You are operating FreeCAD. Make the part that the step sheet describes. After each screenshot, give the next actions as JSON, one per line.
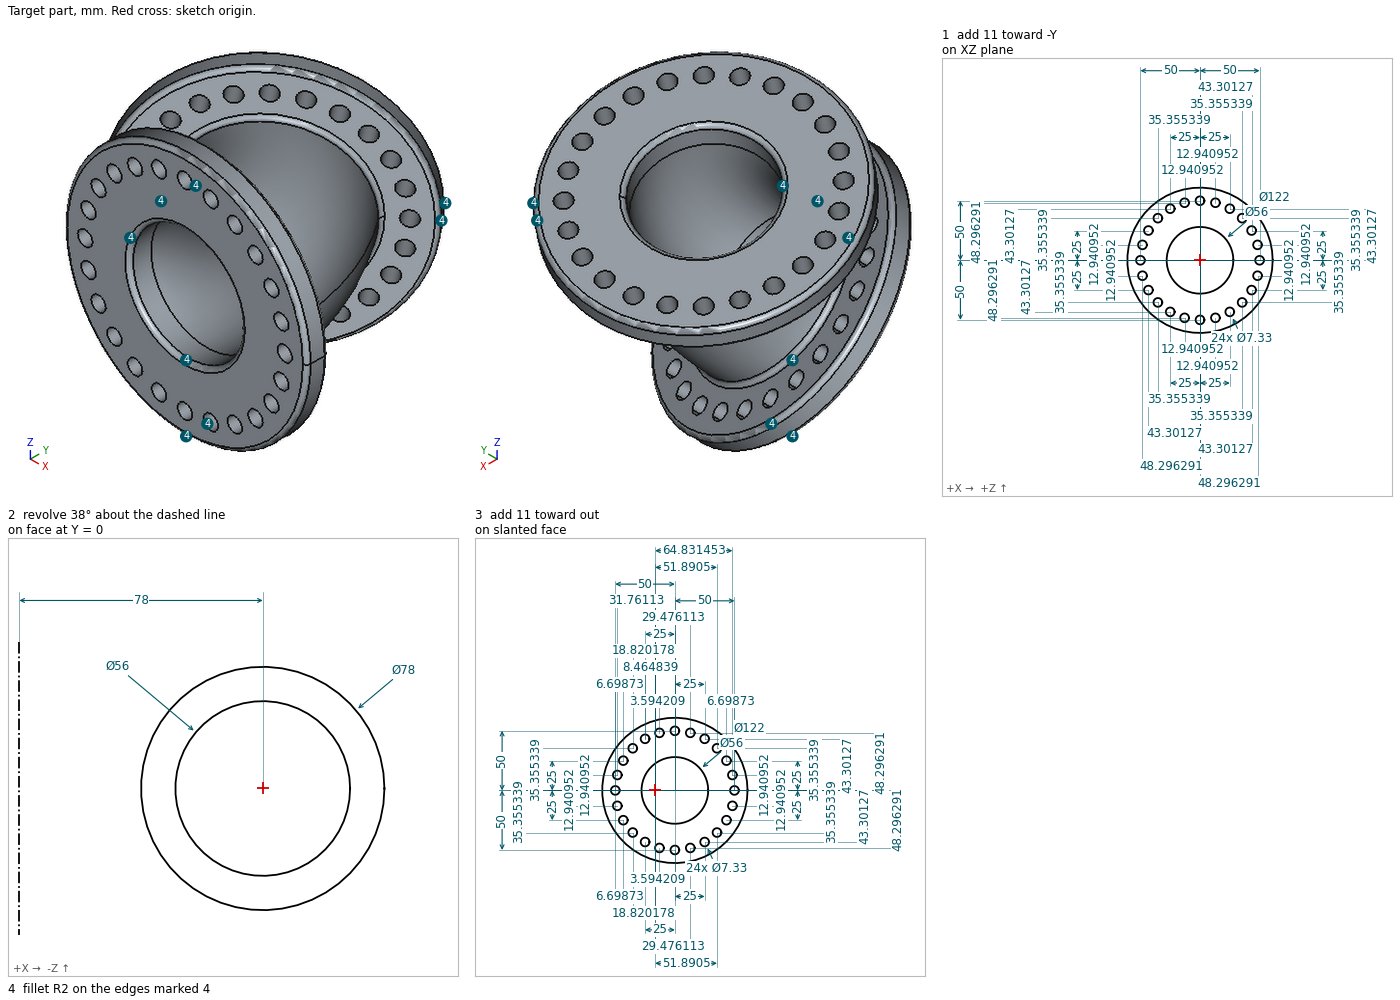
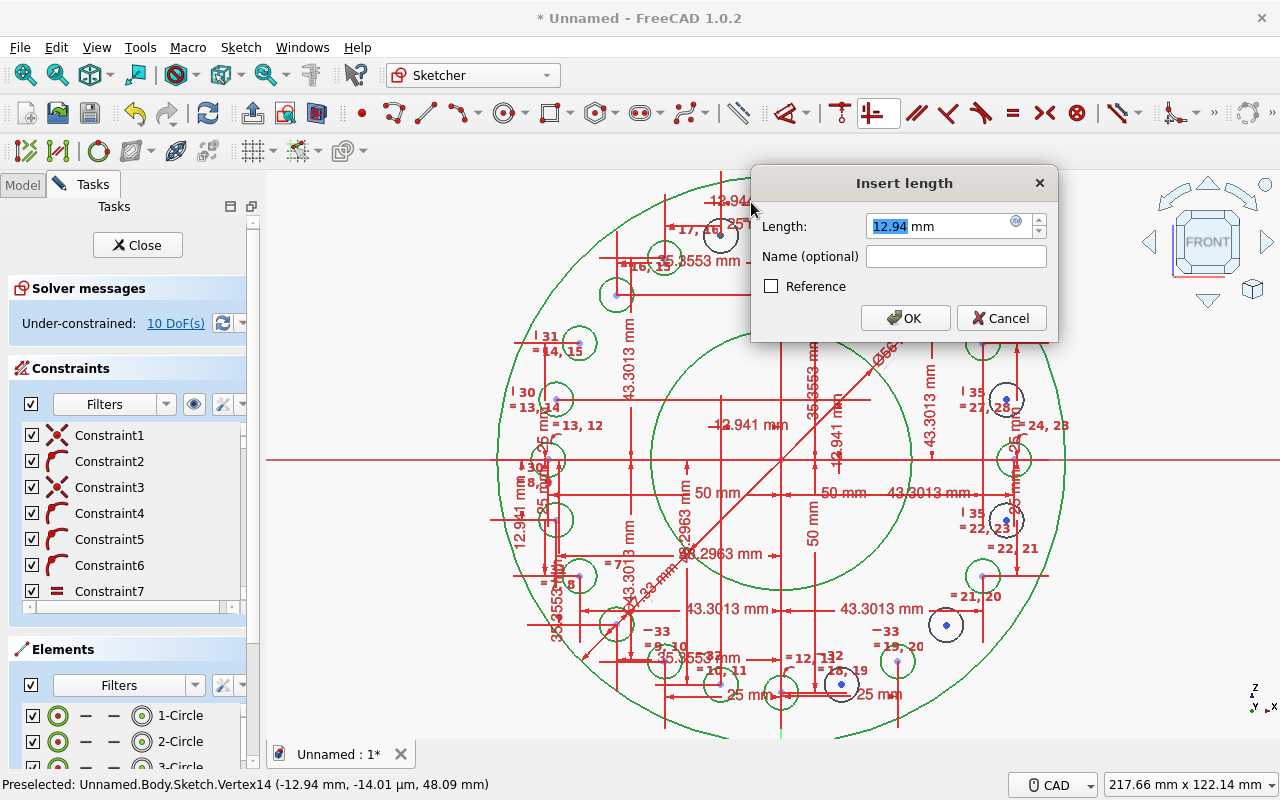
{"action": "type", "text": "12.940952"}
{"action": "key", "text": "Return"}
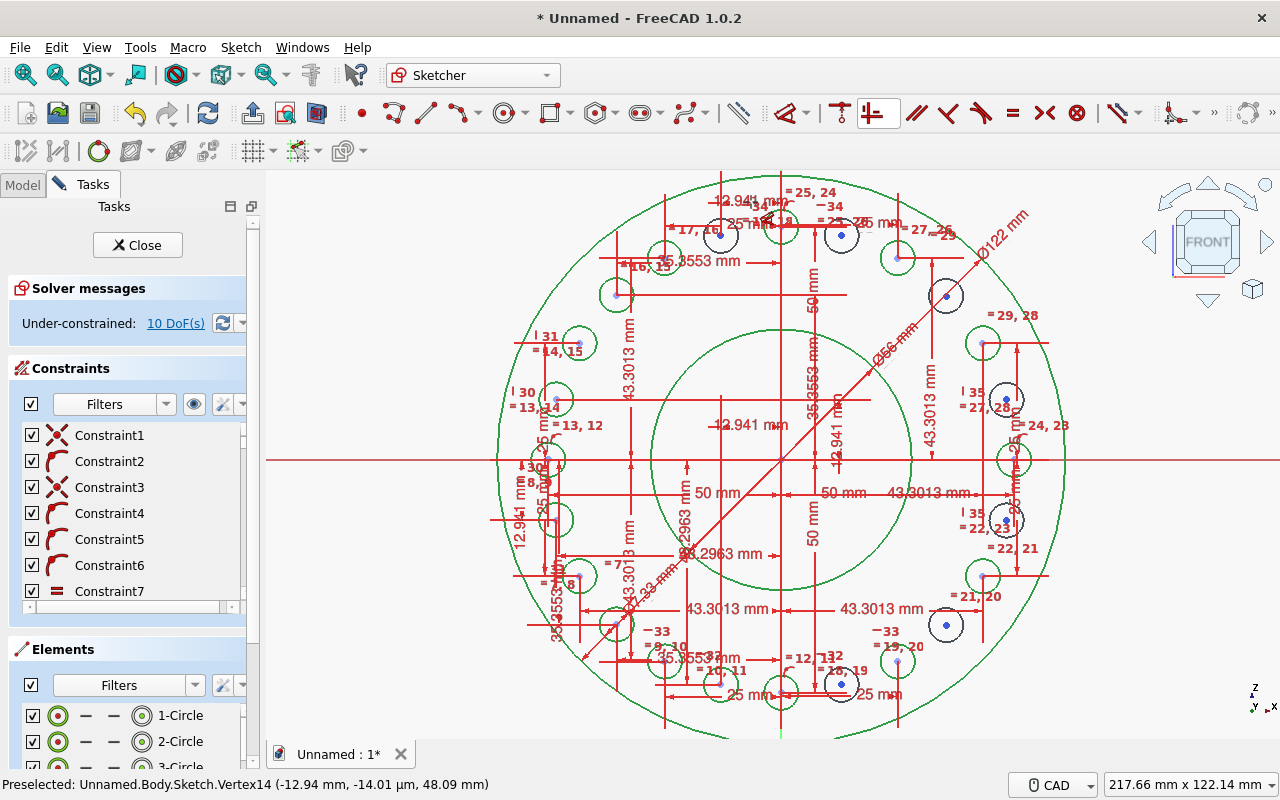
{"action": "left_click", "coordinate": [721, 236]}
{"action": "left_click", "coordinate": [687, 296]}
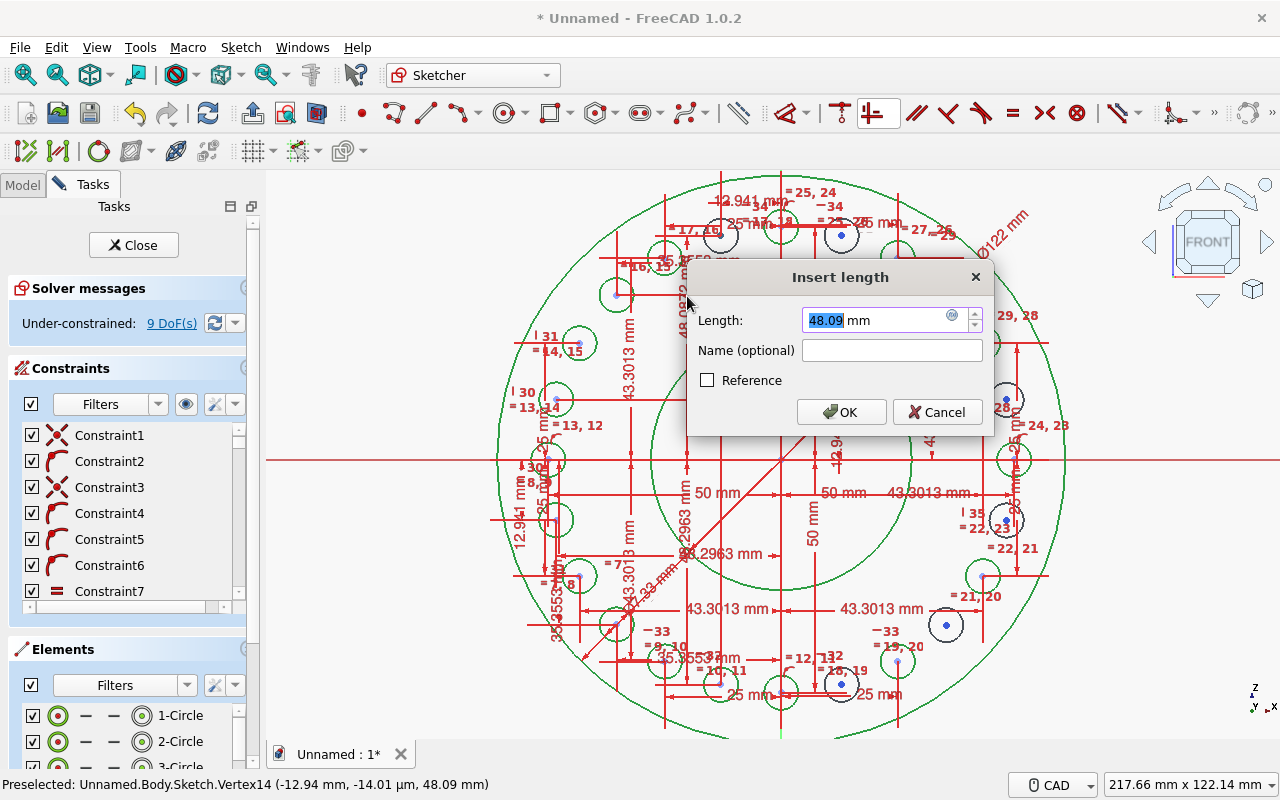
{"action": "type", "text": "48.296291"}
{"action": "key", "text": "Return"}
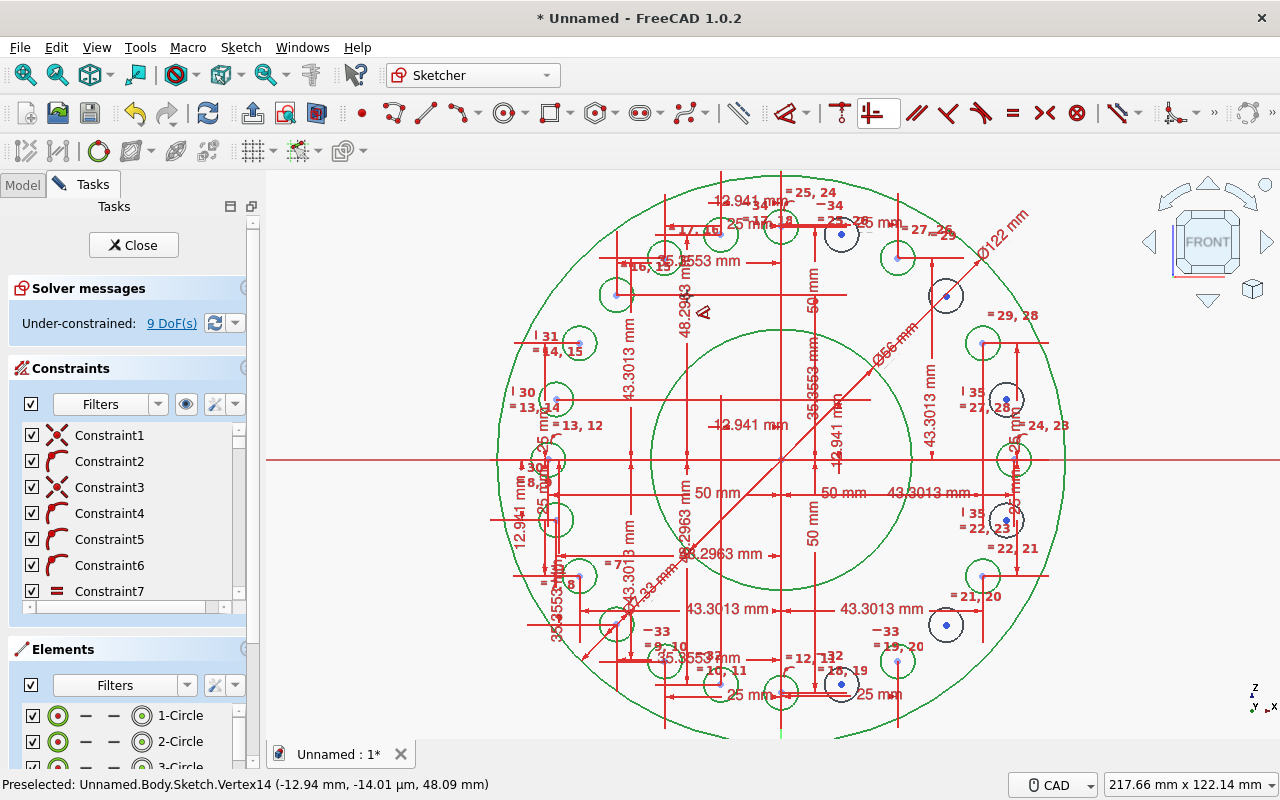
{"action": "left_click", "coordinate": [842, 685]}
{"action": "left_click", "coordinate": [811, 402]}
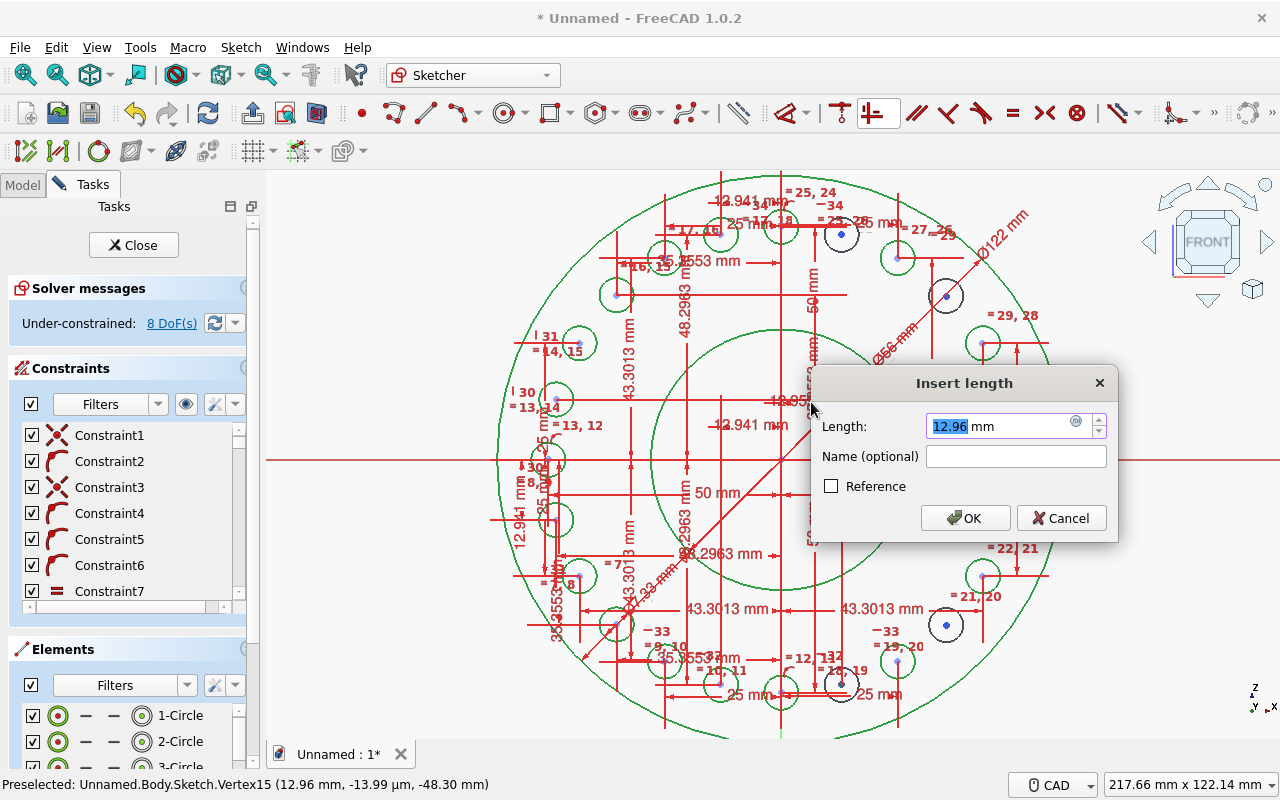
{"action": "type", "text": "12.940952"}
{"action": "key", "text": "Return"}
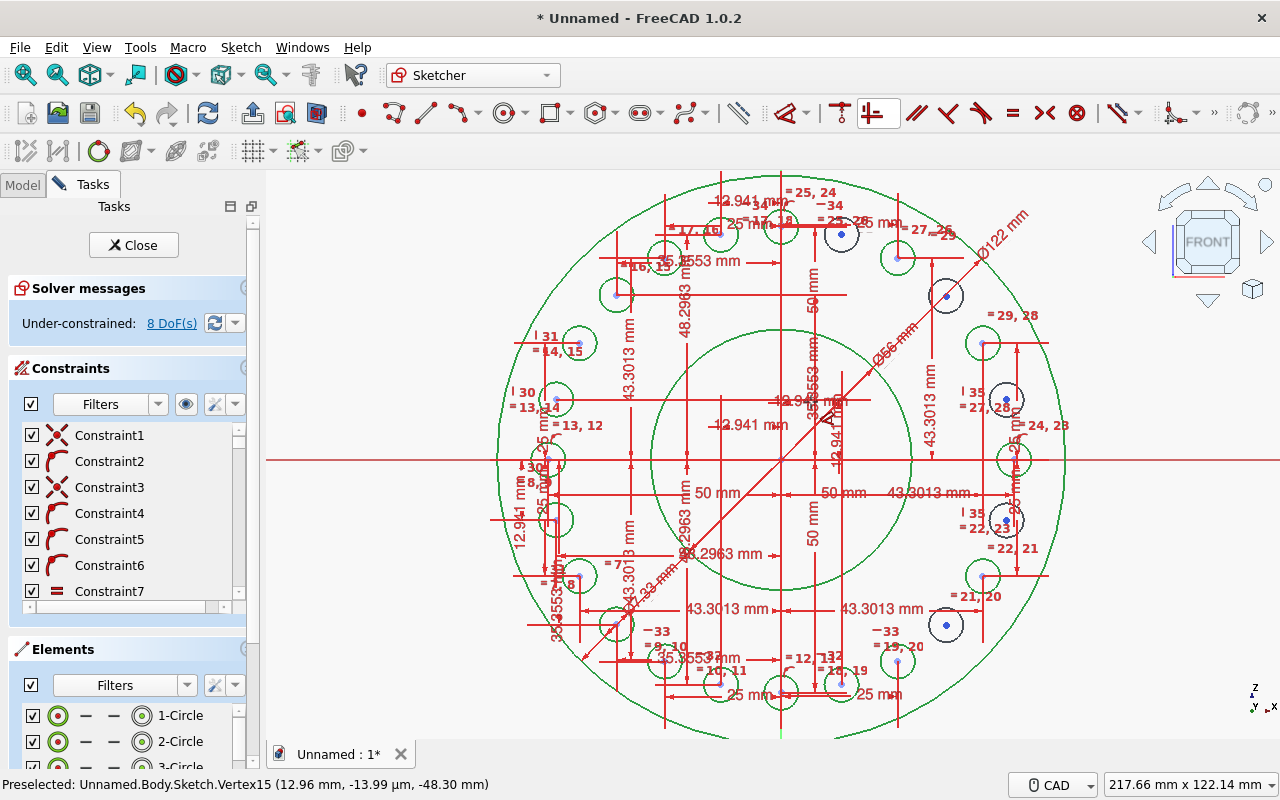
{"action": "left_click", "coordinate": [946, 625]}
{"action": "left_click", "coordinate": [864, 659]}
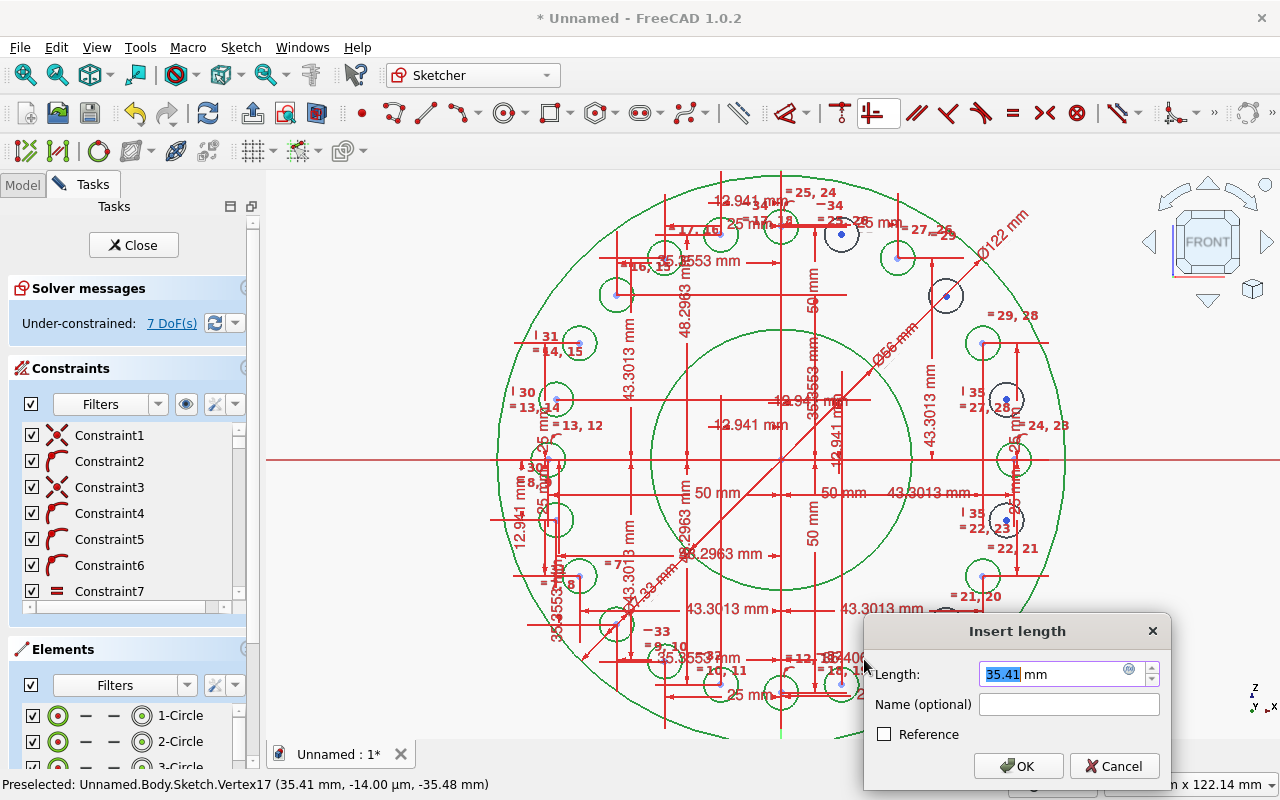
{"action": "type", "text": "35.355339"}
{"action": "key", "text": "Return"}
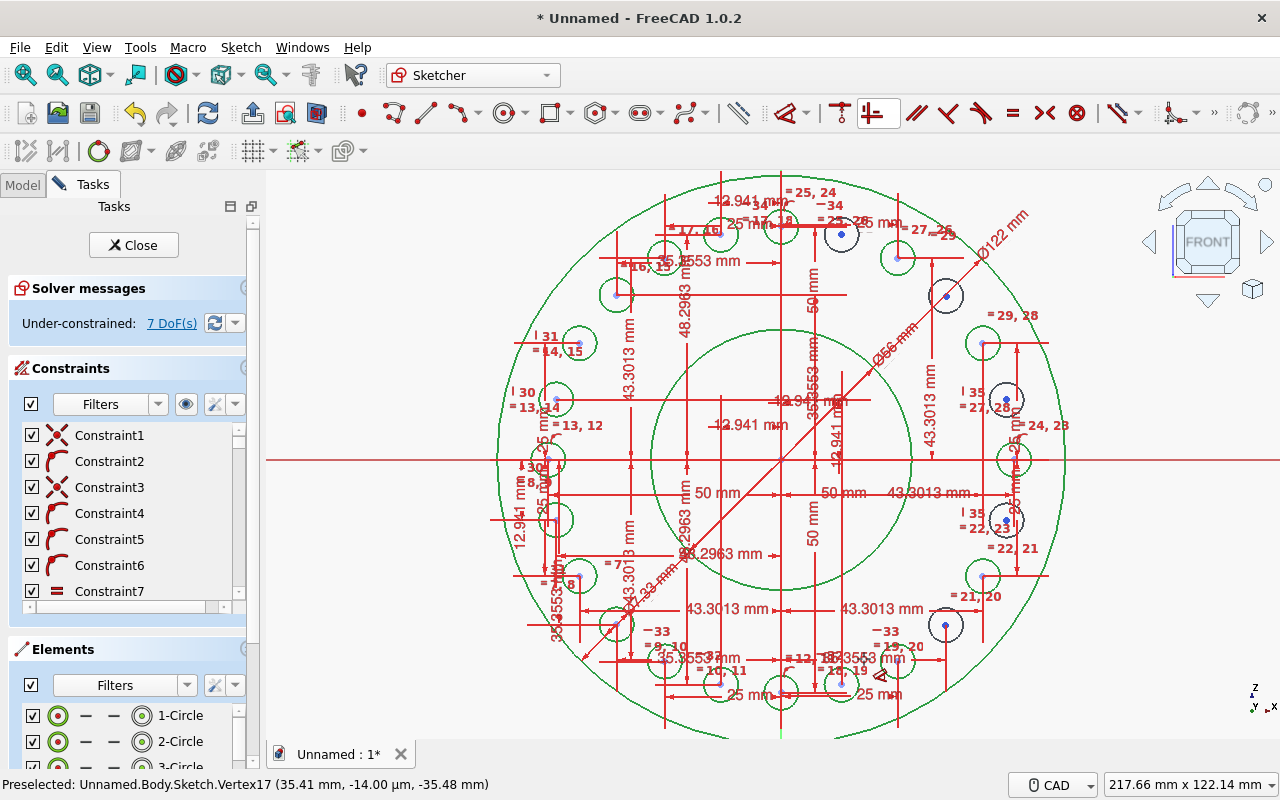
{"action": "left_click", "coordinate": [946, 625]}
{"action": "left_click", "coordinate": [980, 542]}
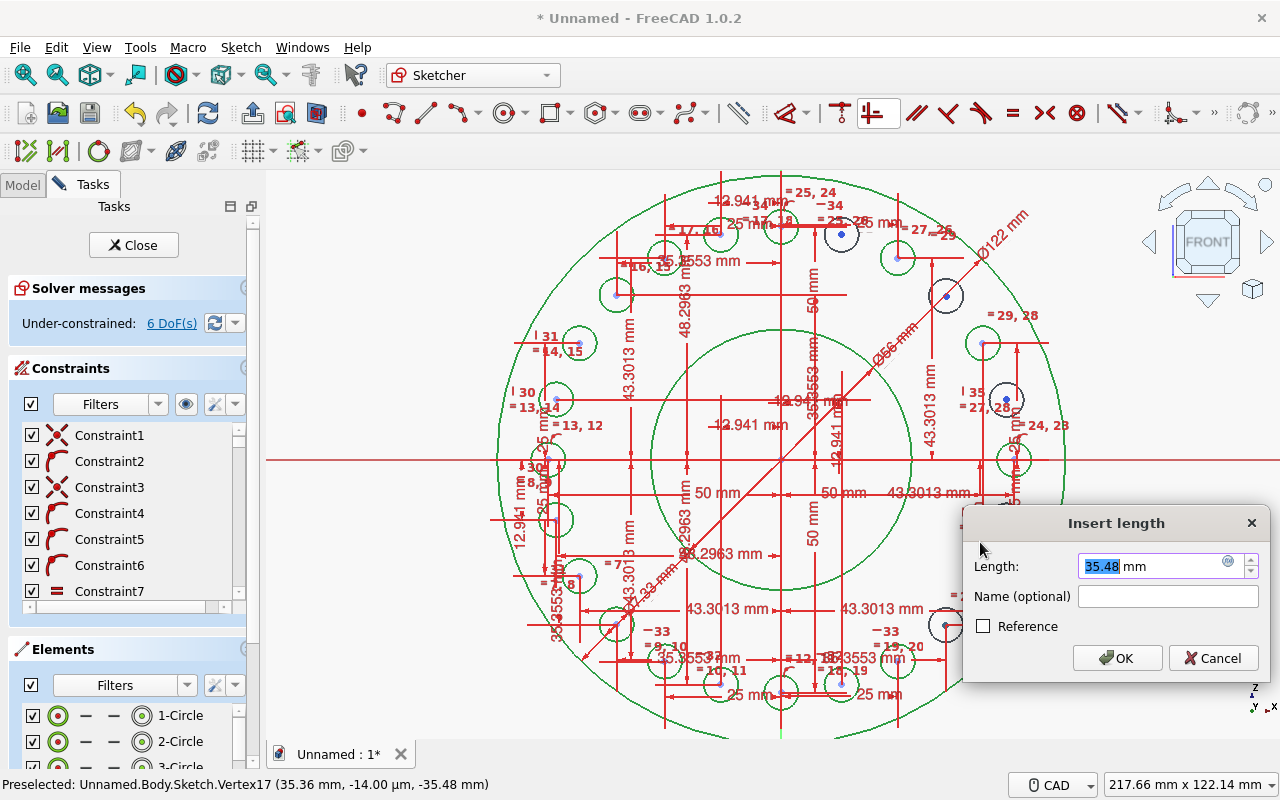
{"action": "type", "text": "35.355339"}
{"action": "key", "text": "Return"}